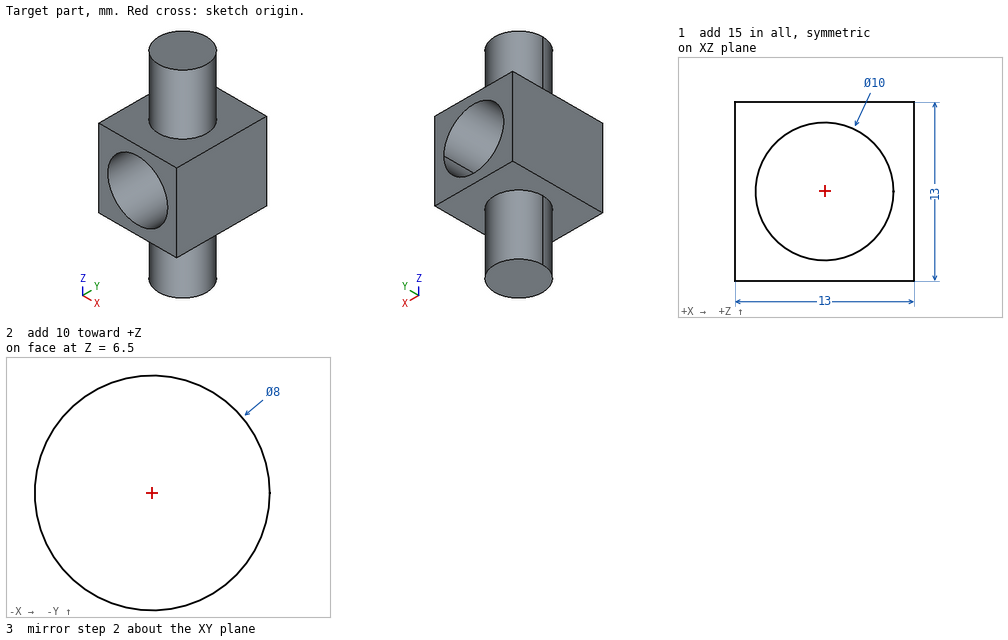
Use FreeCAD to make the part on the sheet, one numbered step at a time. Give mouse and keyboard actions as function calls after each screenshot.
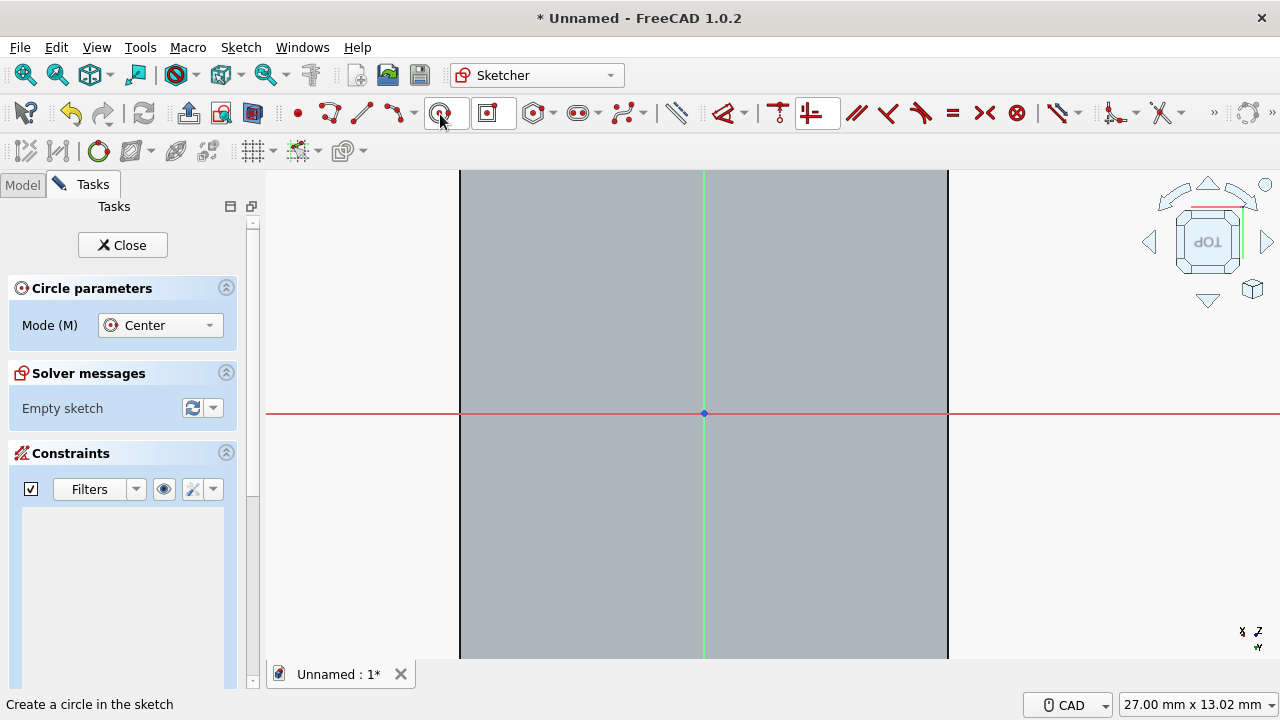
click(704, 414)
move(810, 307)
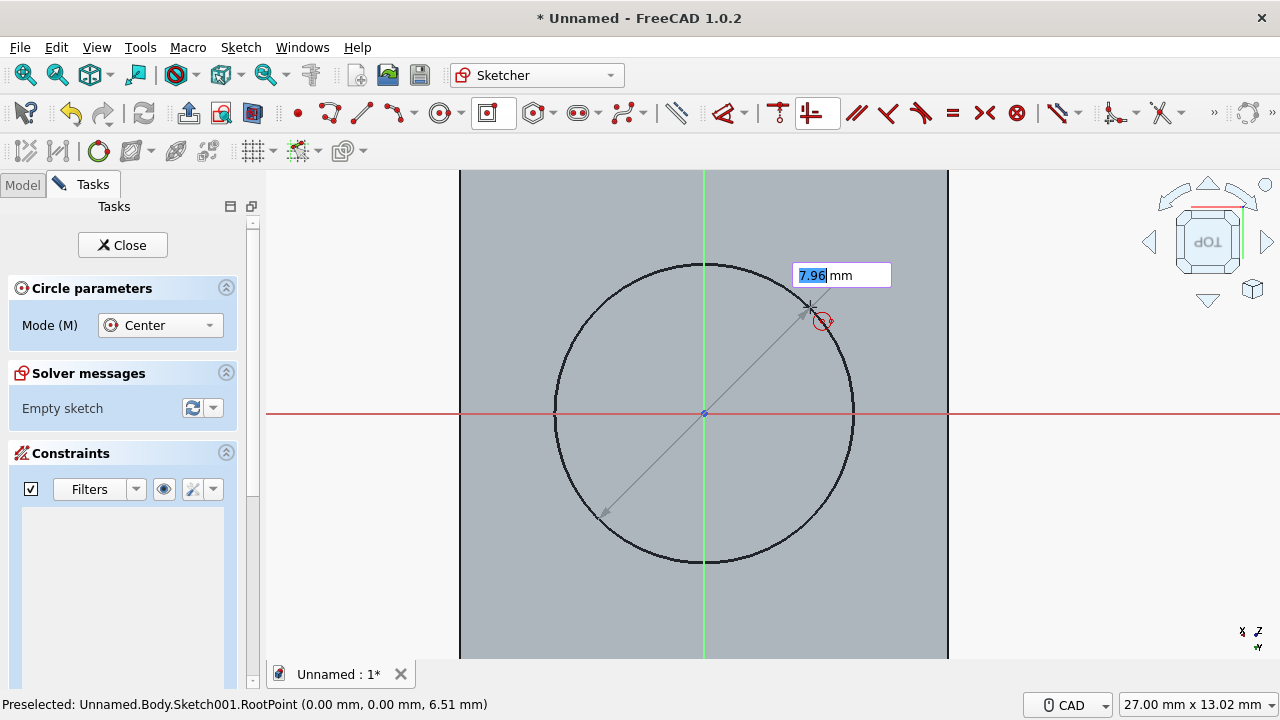
text(8)
key(Return)
key(Escape)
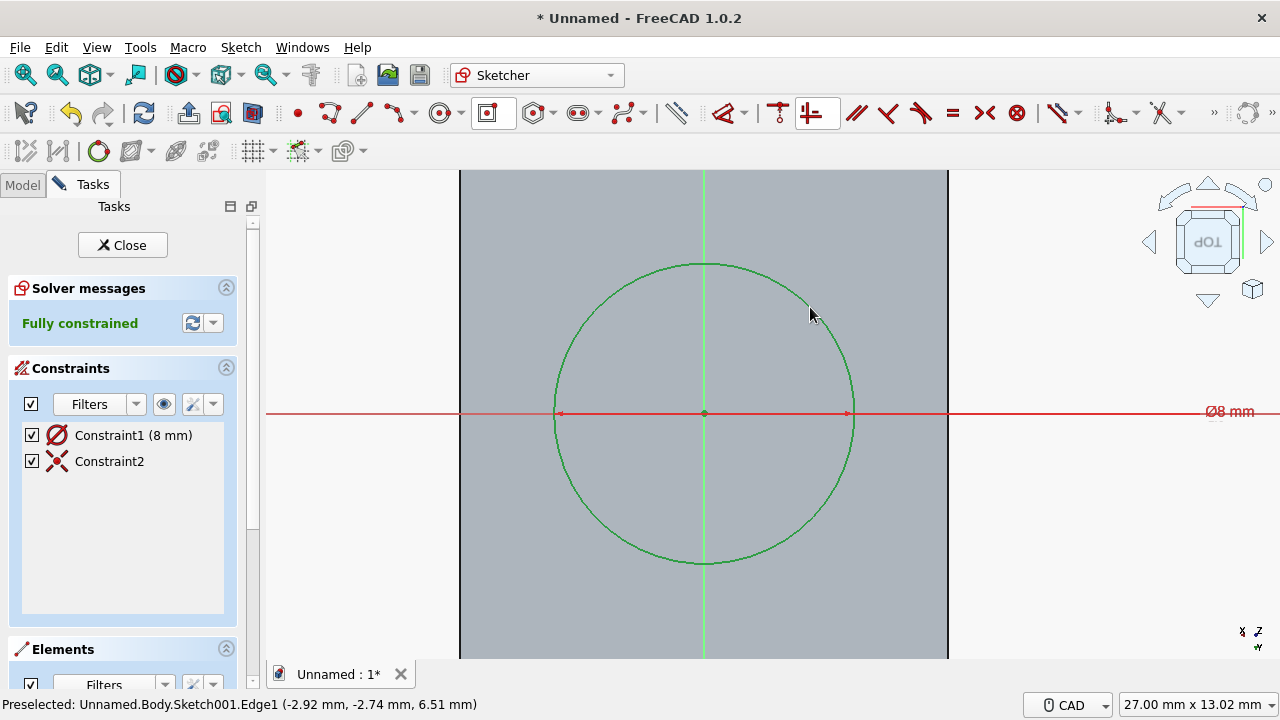
click(123, 245)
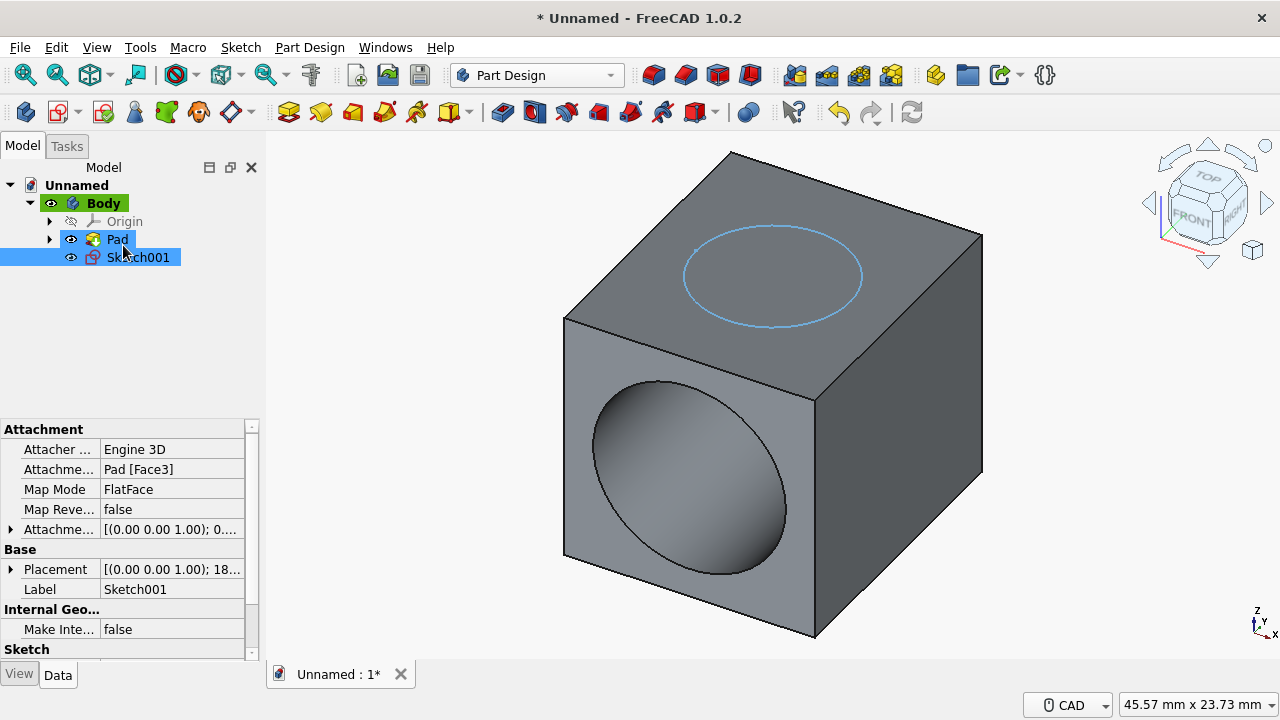
click(290, 112)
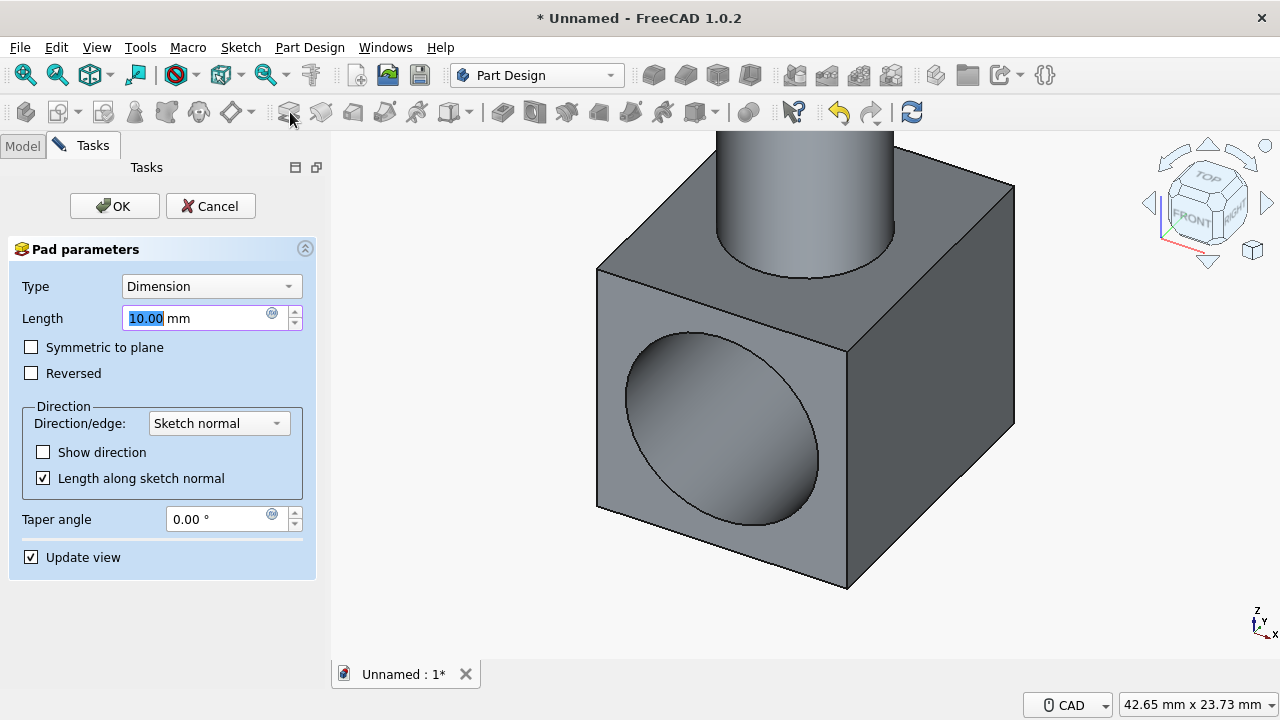
text(10)
key(Tab)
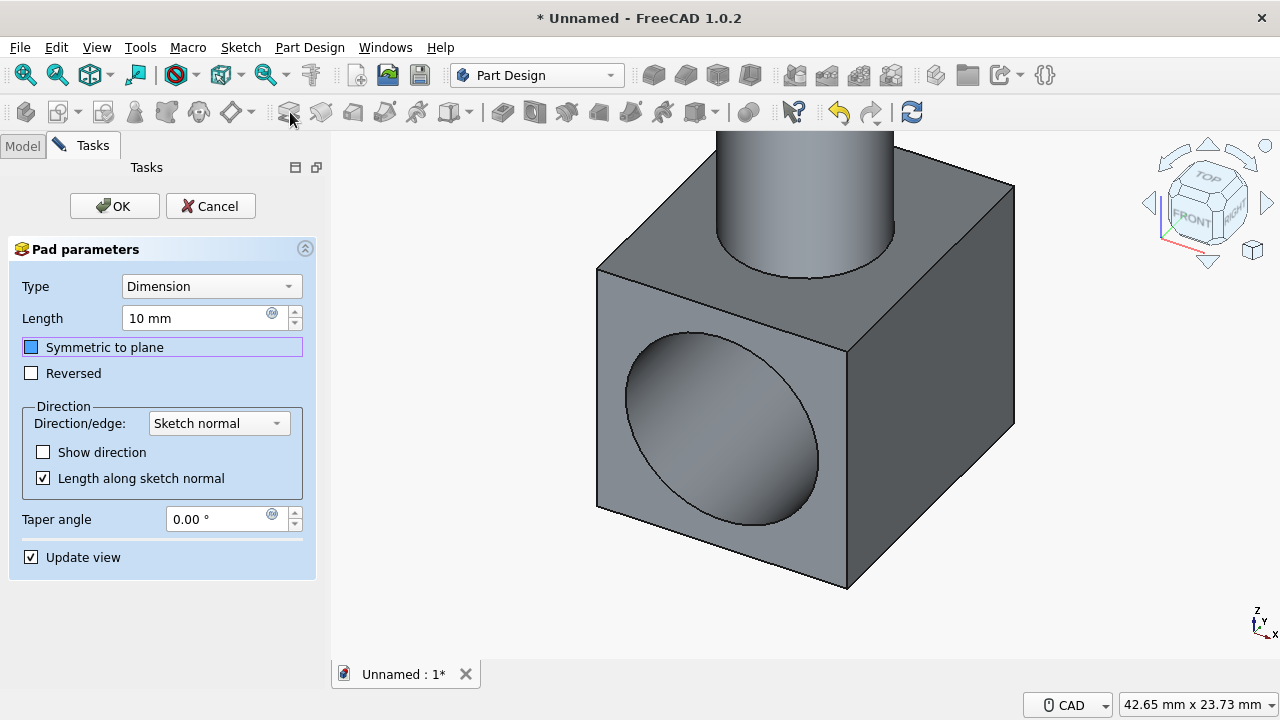
click(115, 206)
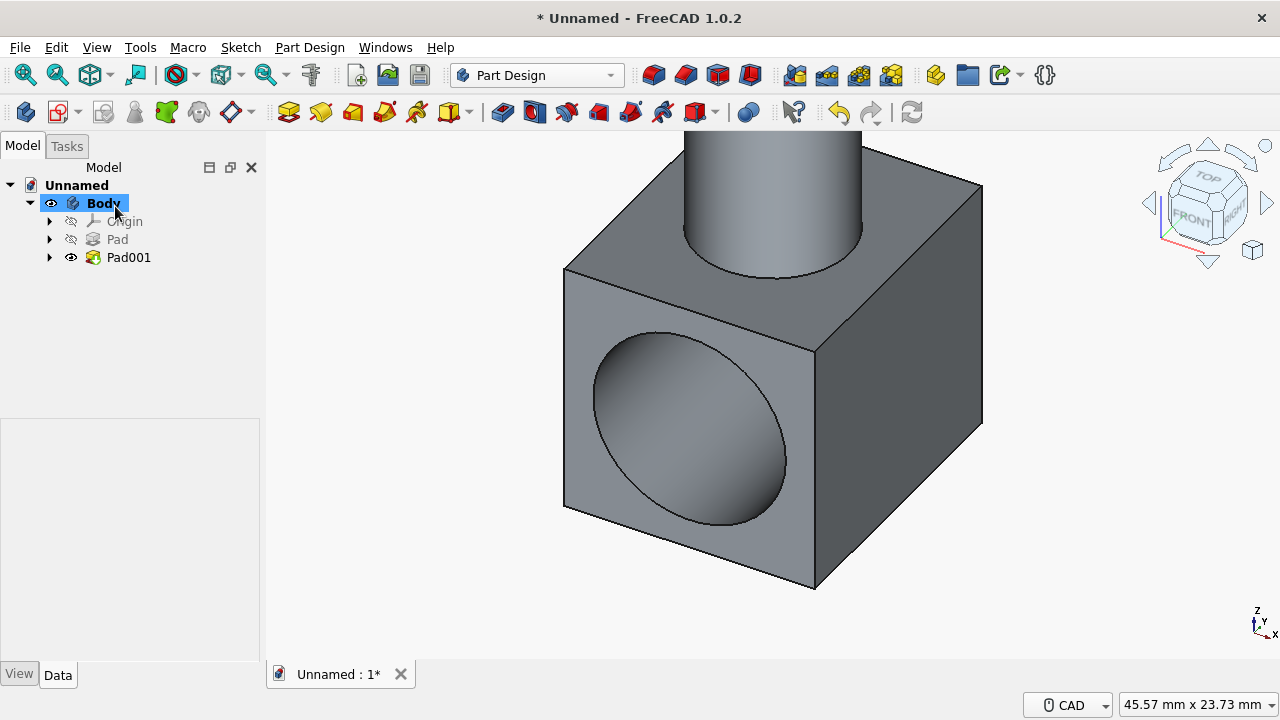
click(26, 76)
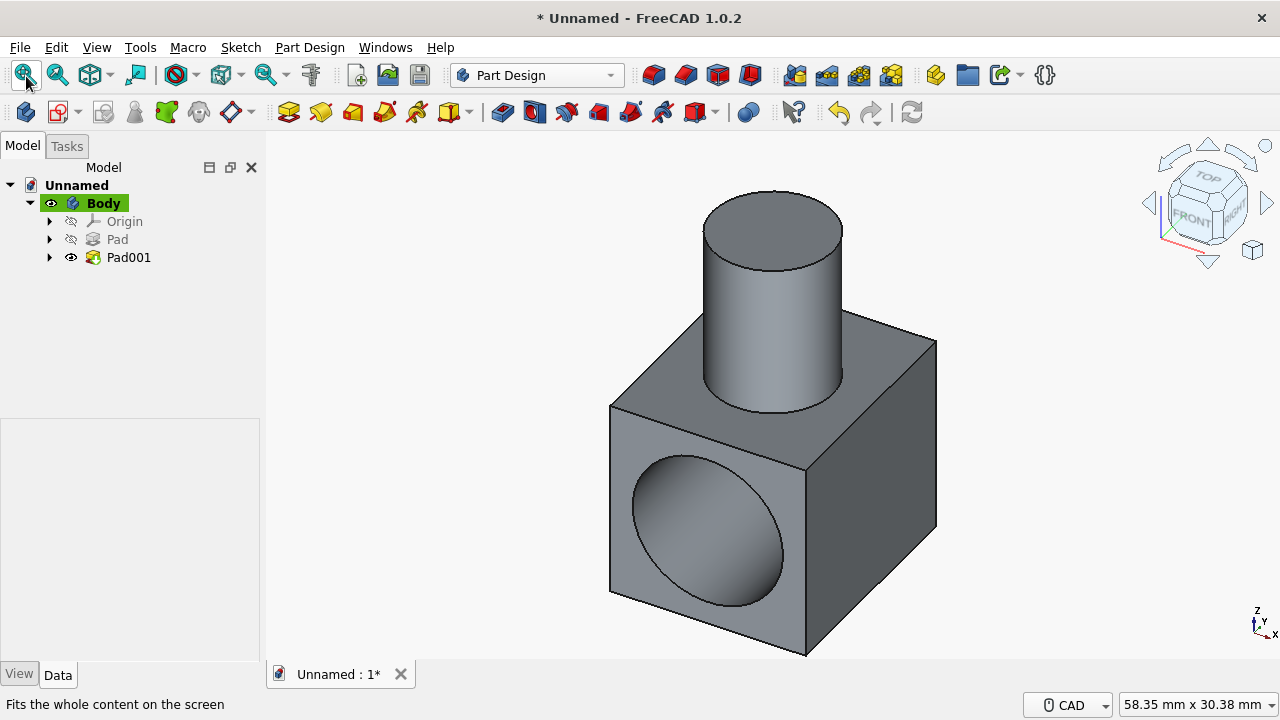
click(116, 257)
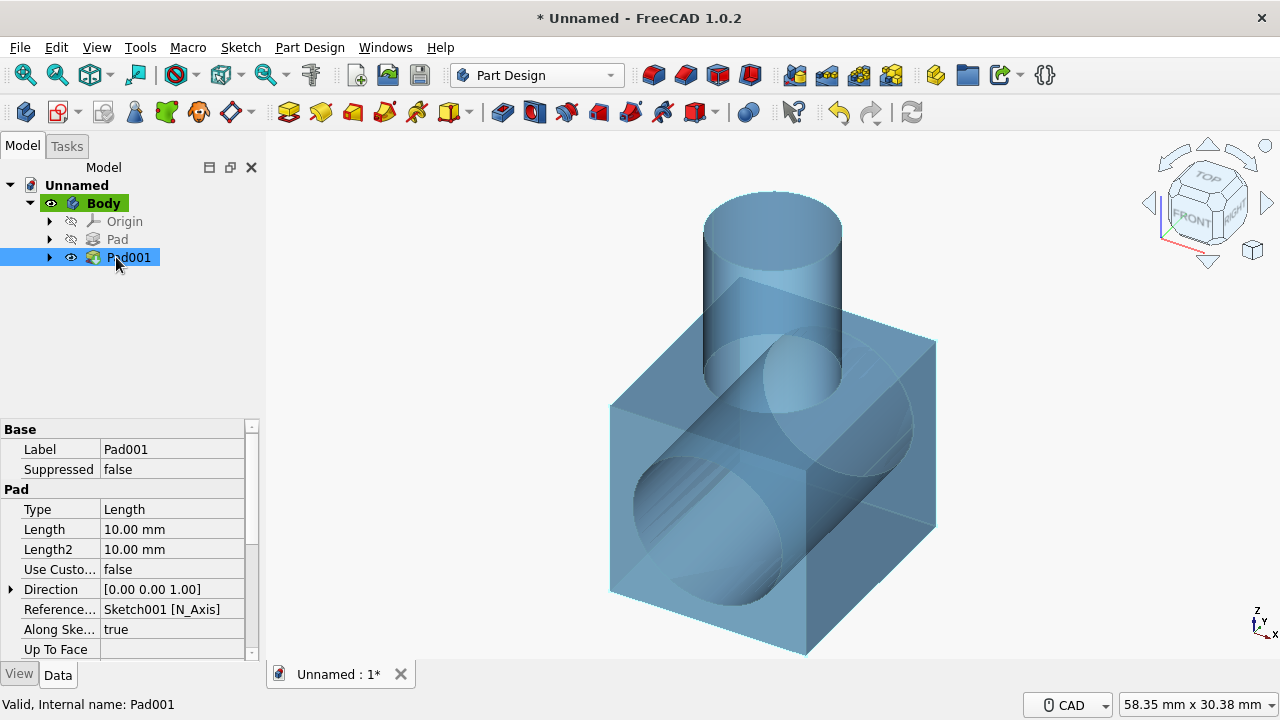
click(796, 76)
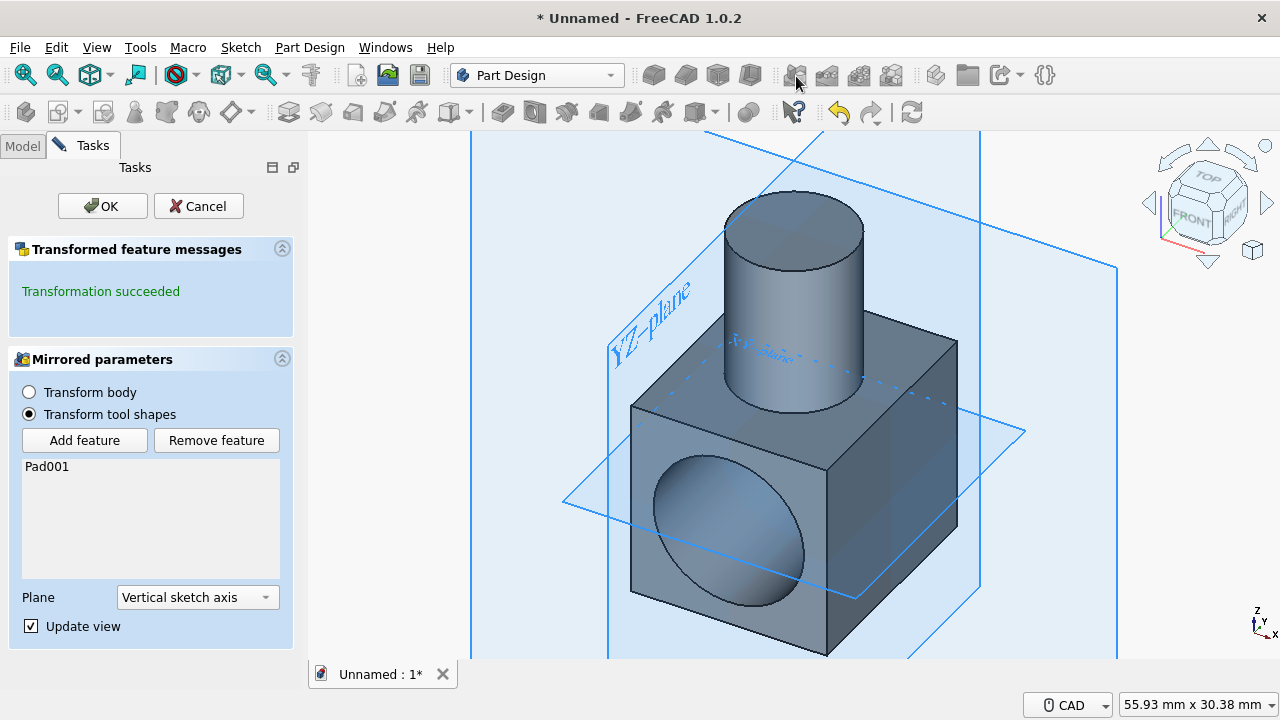
click(198, 598)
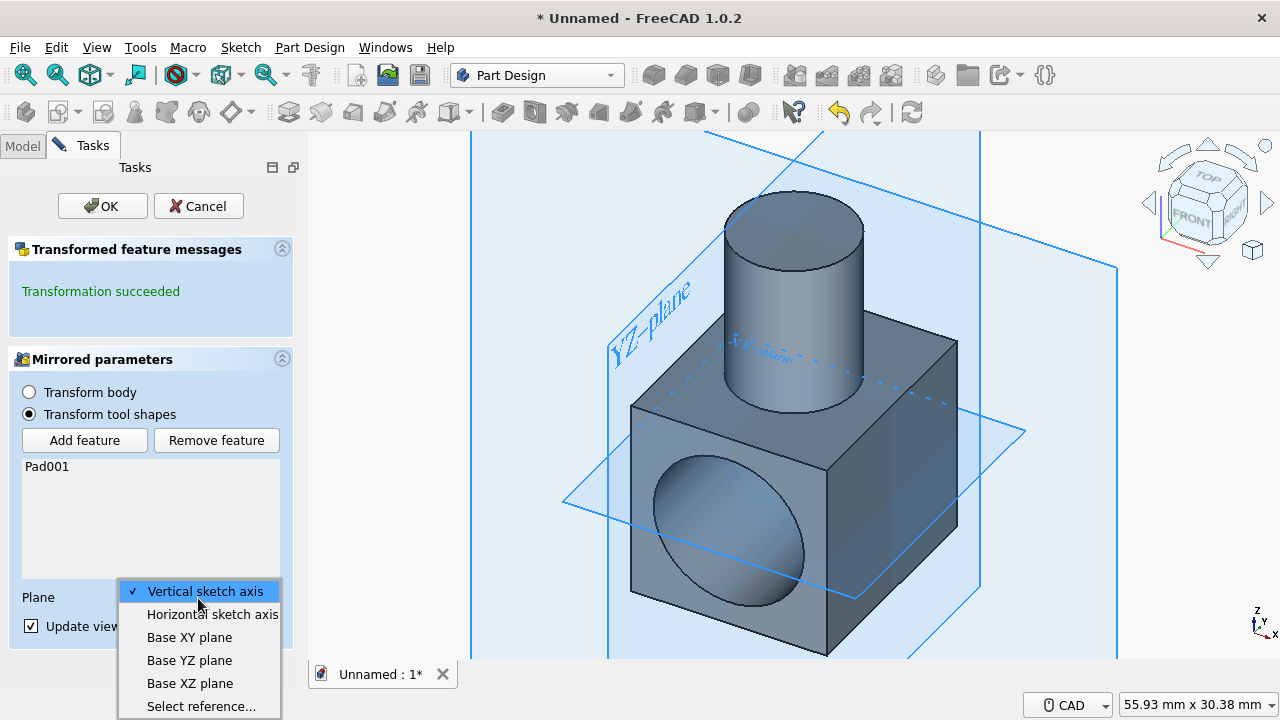
click(198, 638)